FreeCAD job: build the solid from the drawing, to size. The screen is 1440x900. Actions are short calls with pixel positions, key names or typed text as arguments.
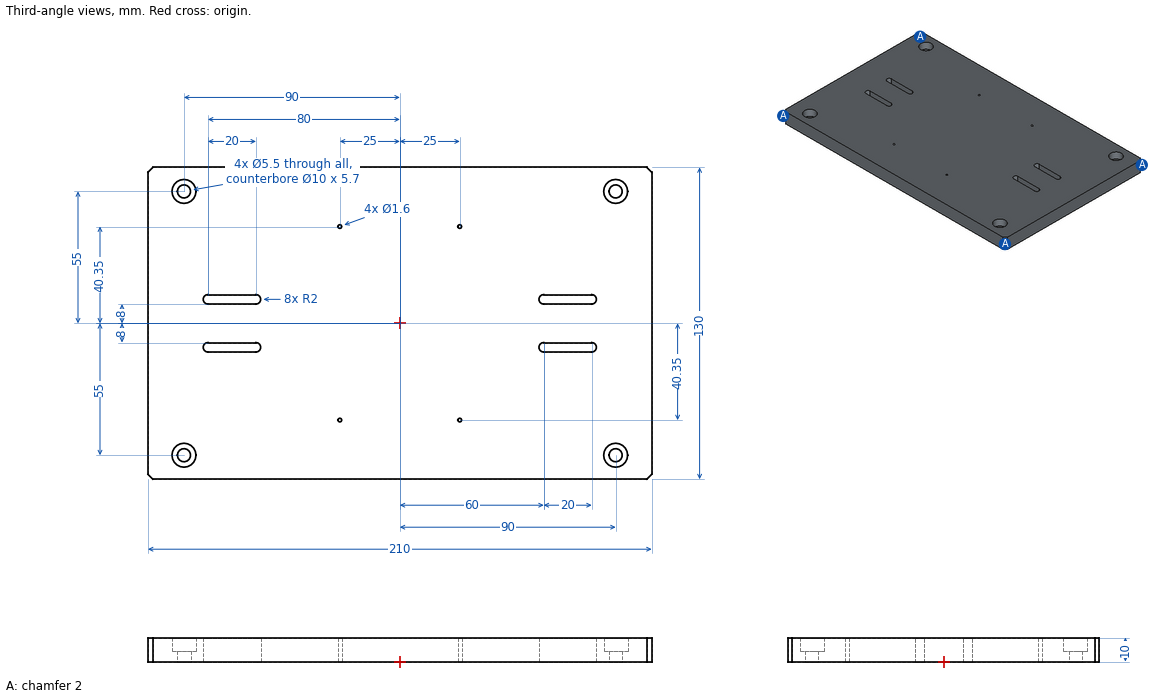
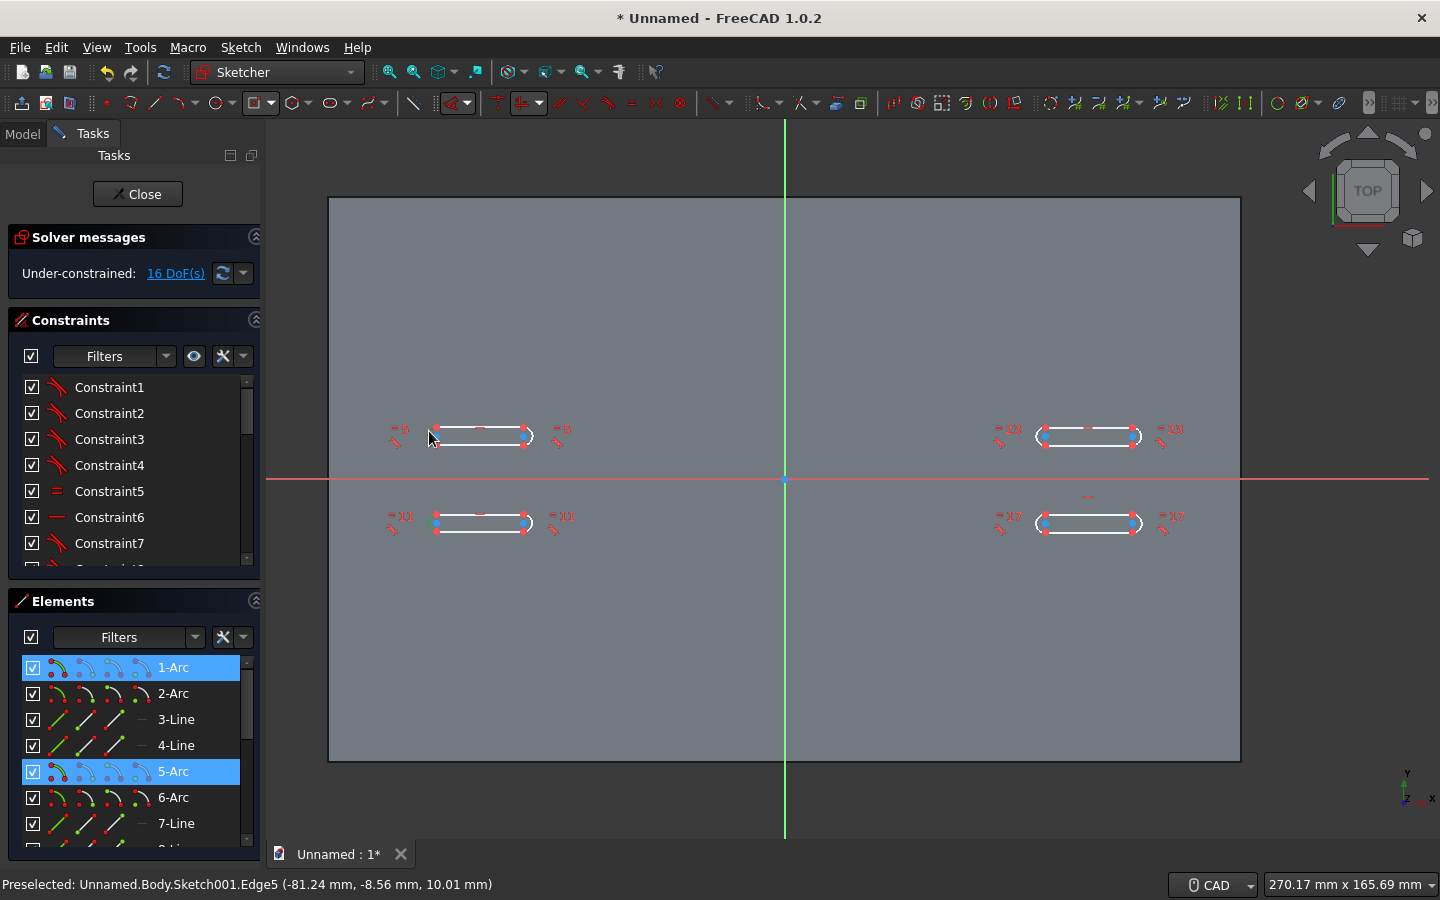
scroll(1038, 518, up, 3)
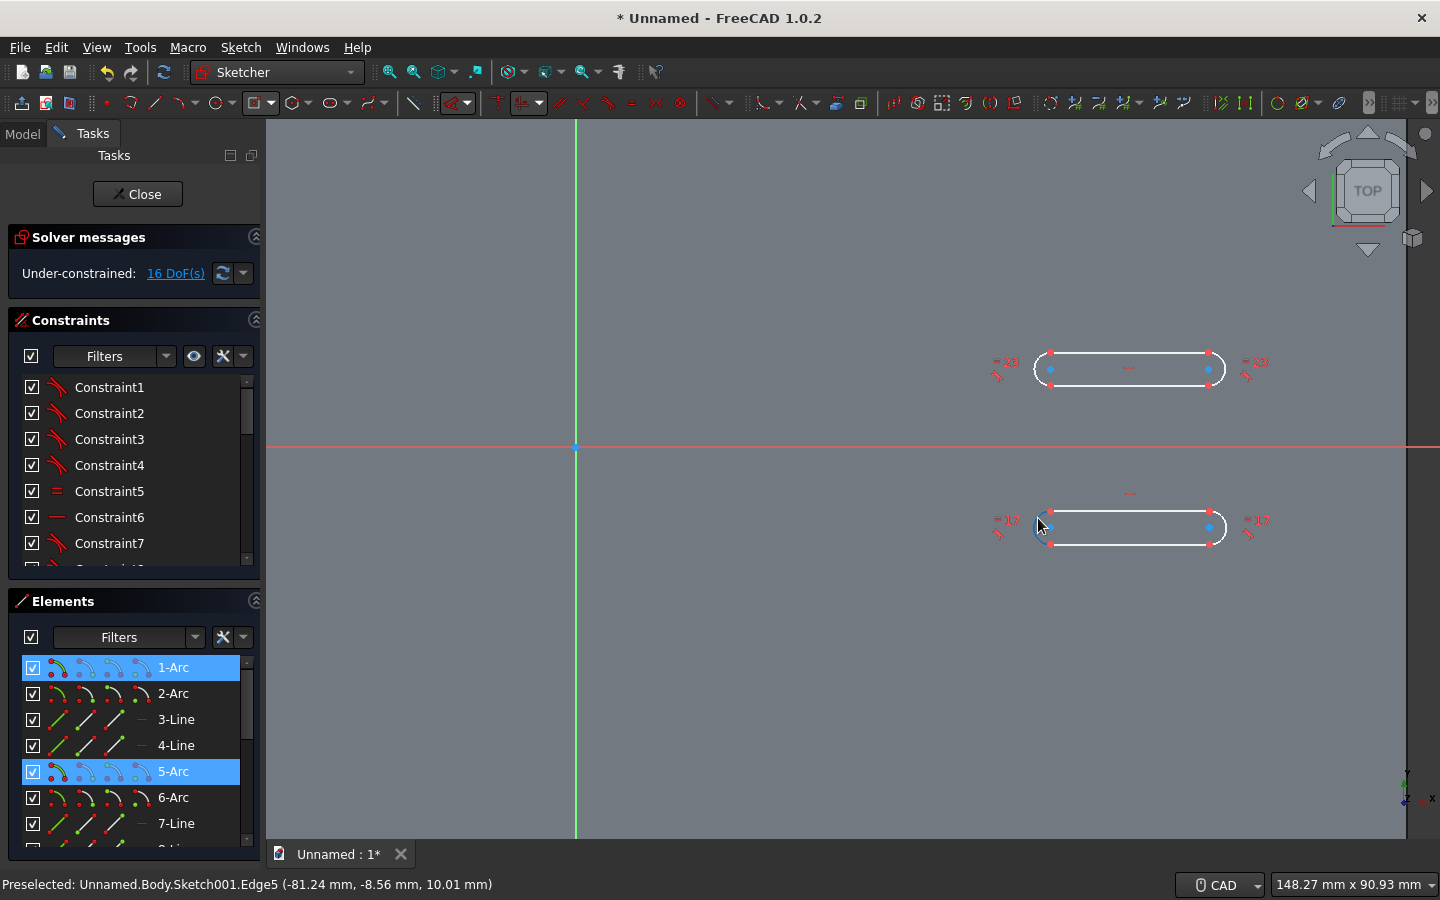
click(1037, 518)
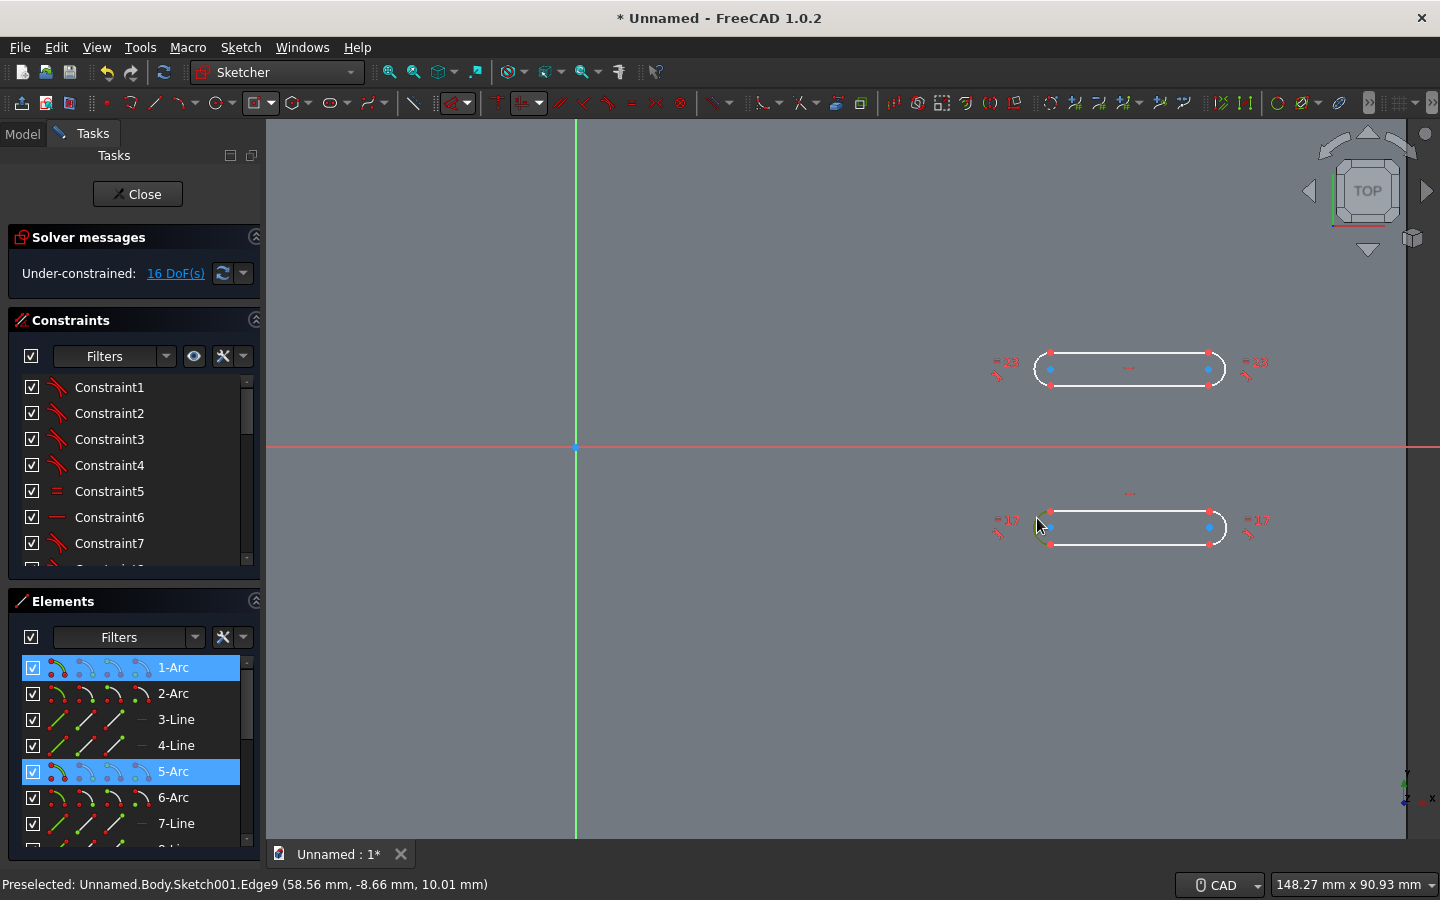
click(1038, 360)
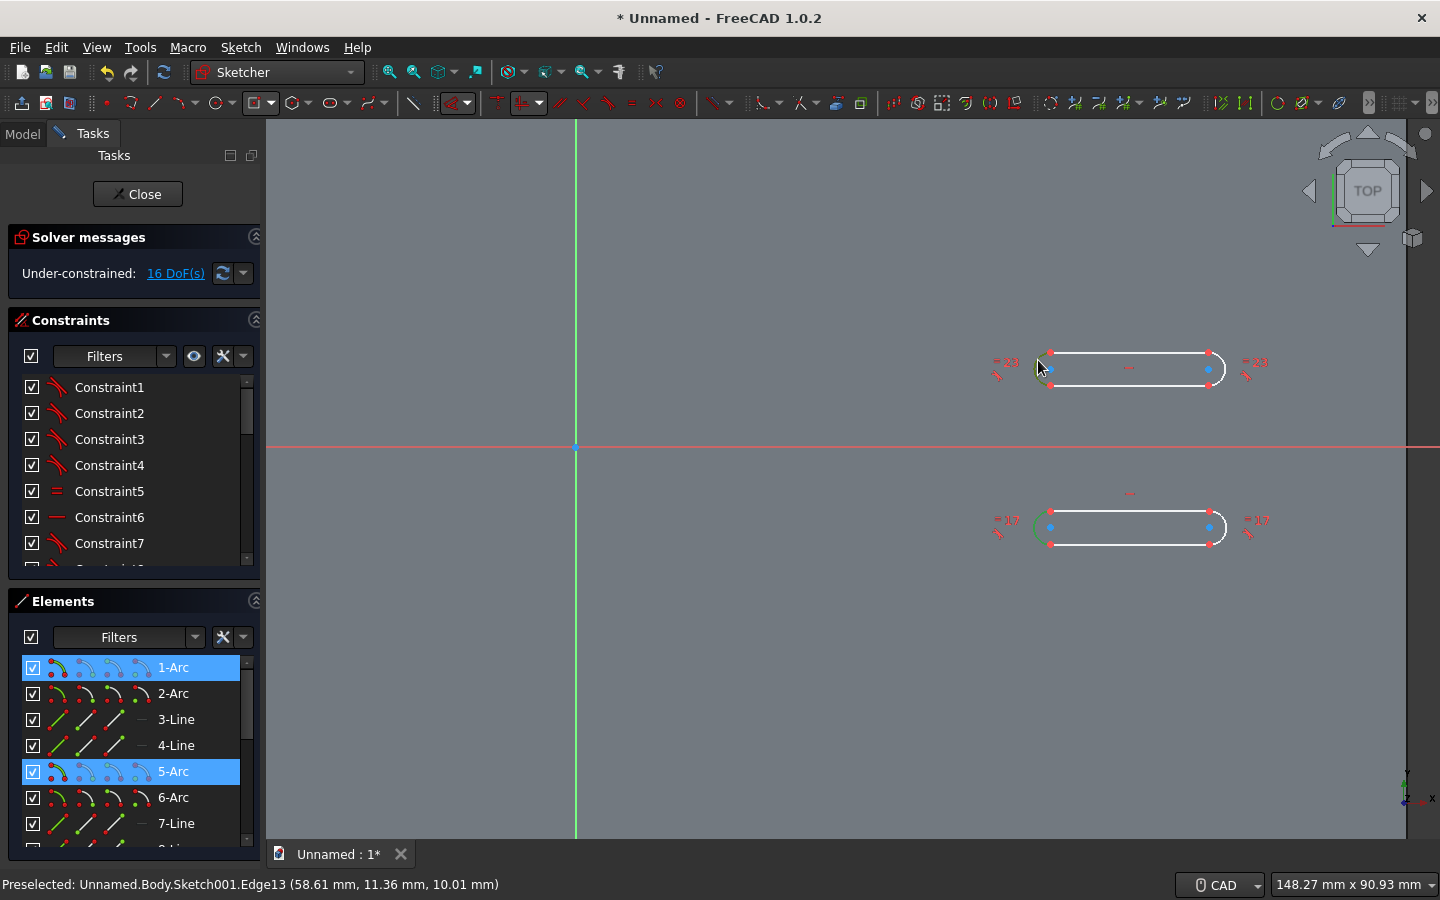
click(632, 104)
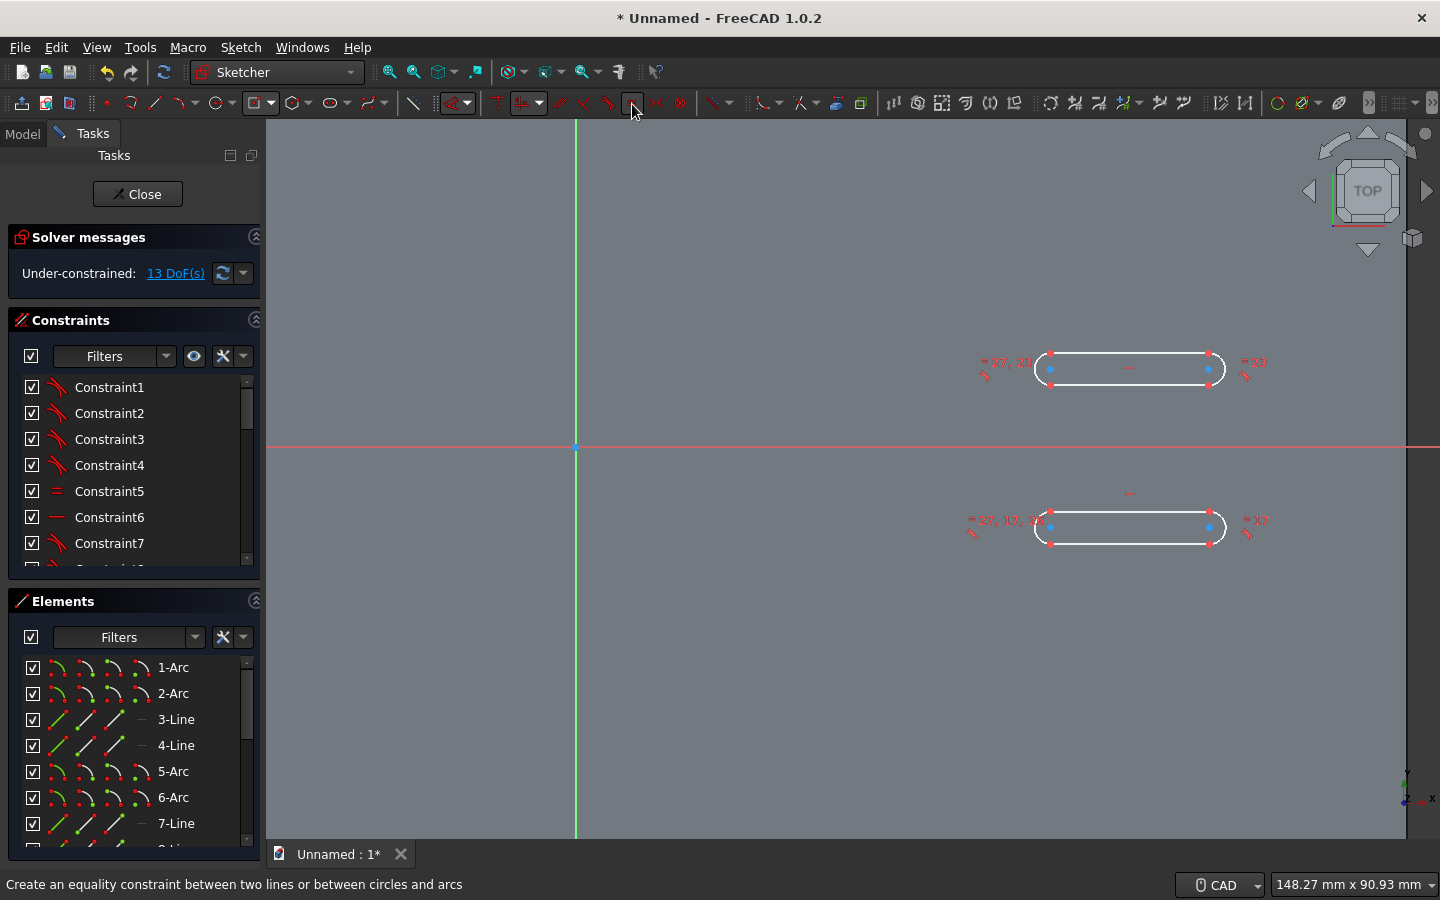
scroll(1039, 518, down, 3)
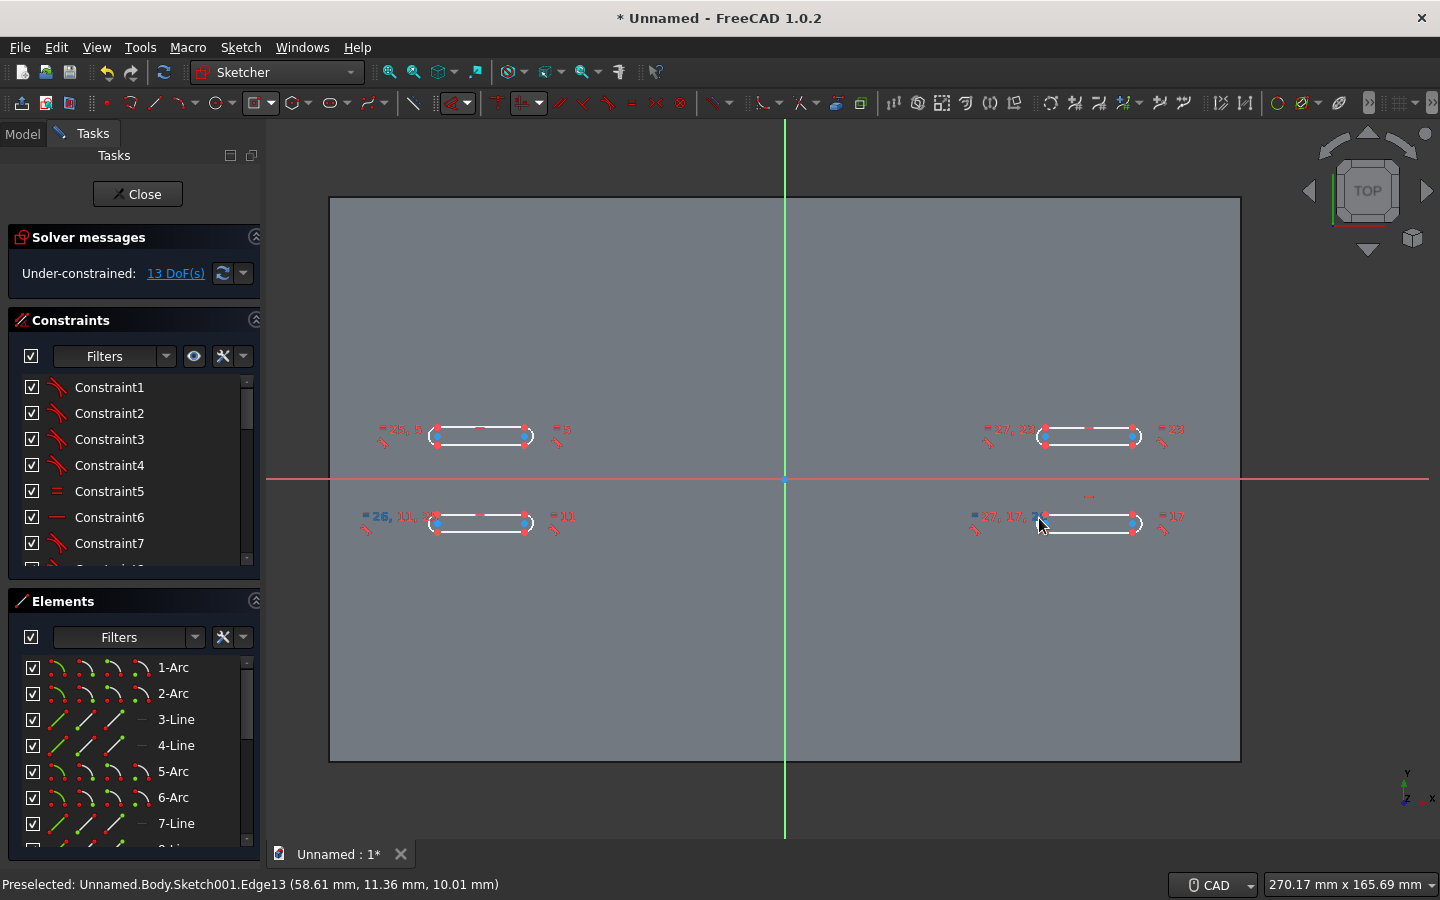
scroll(430, 431, up, 8)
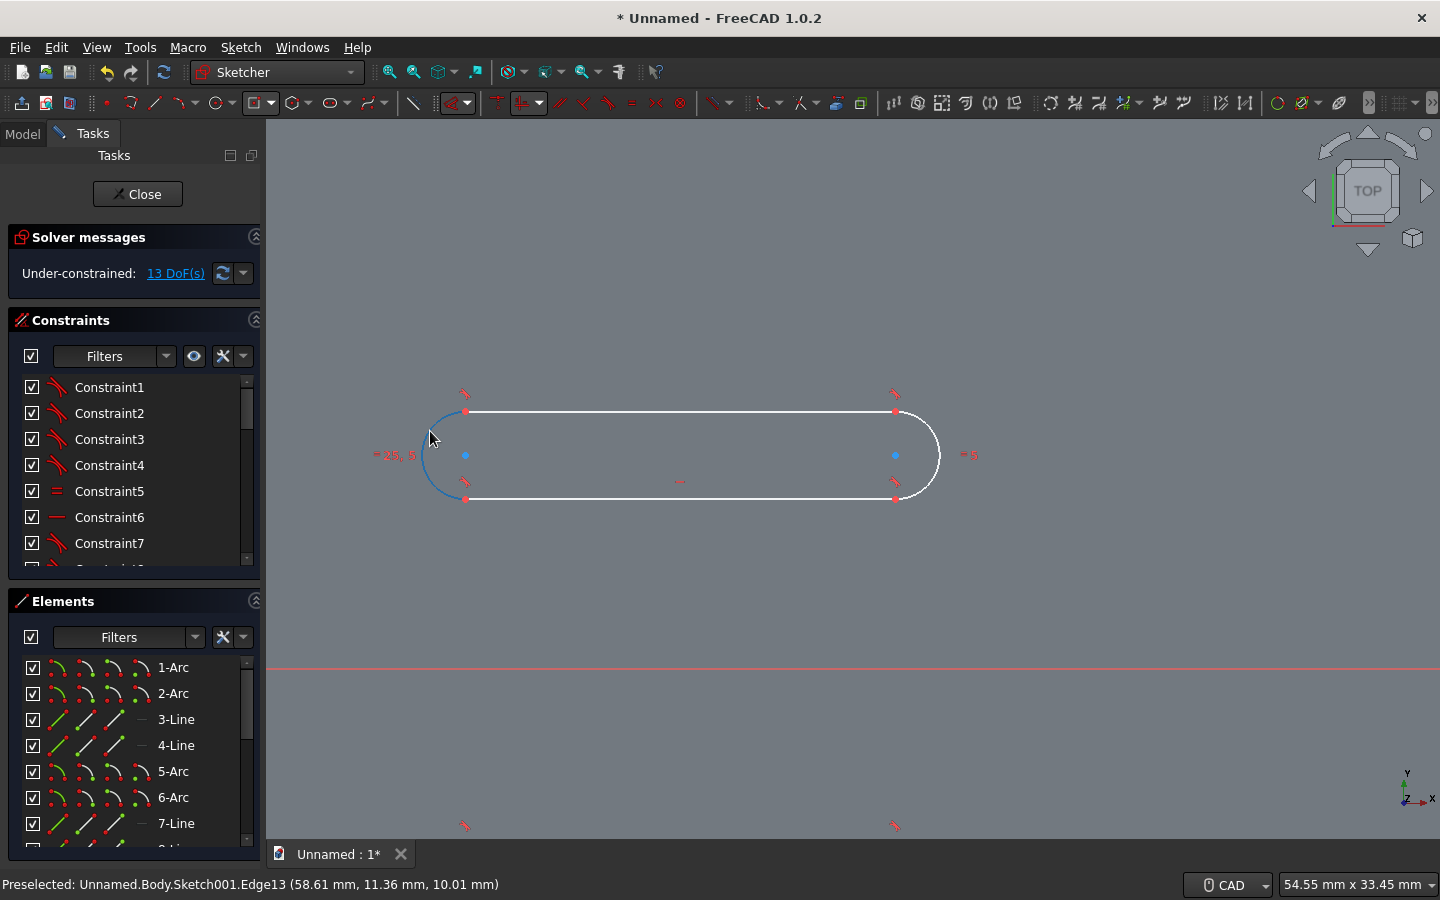
click(431, 430)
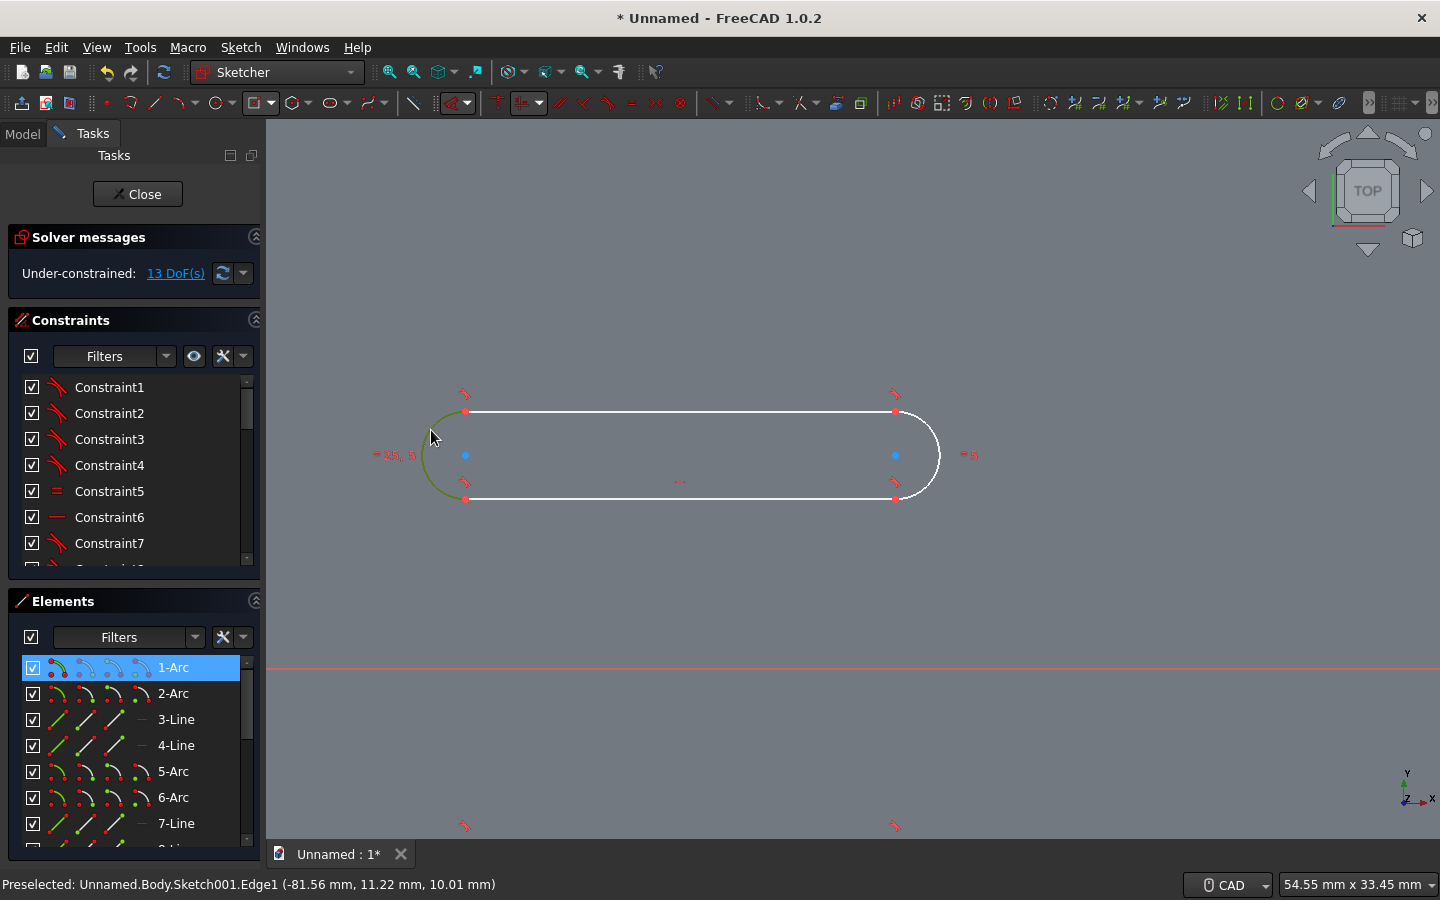
click(470, 104)